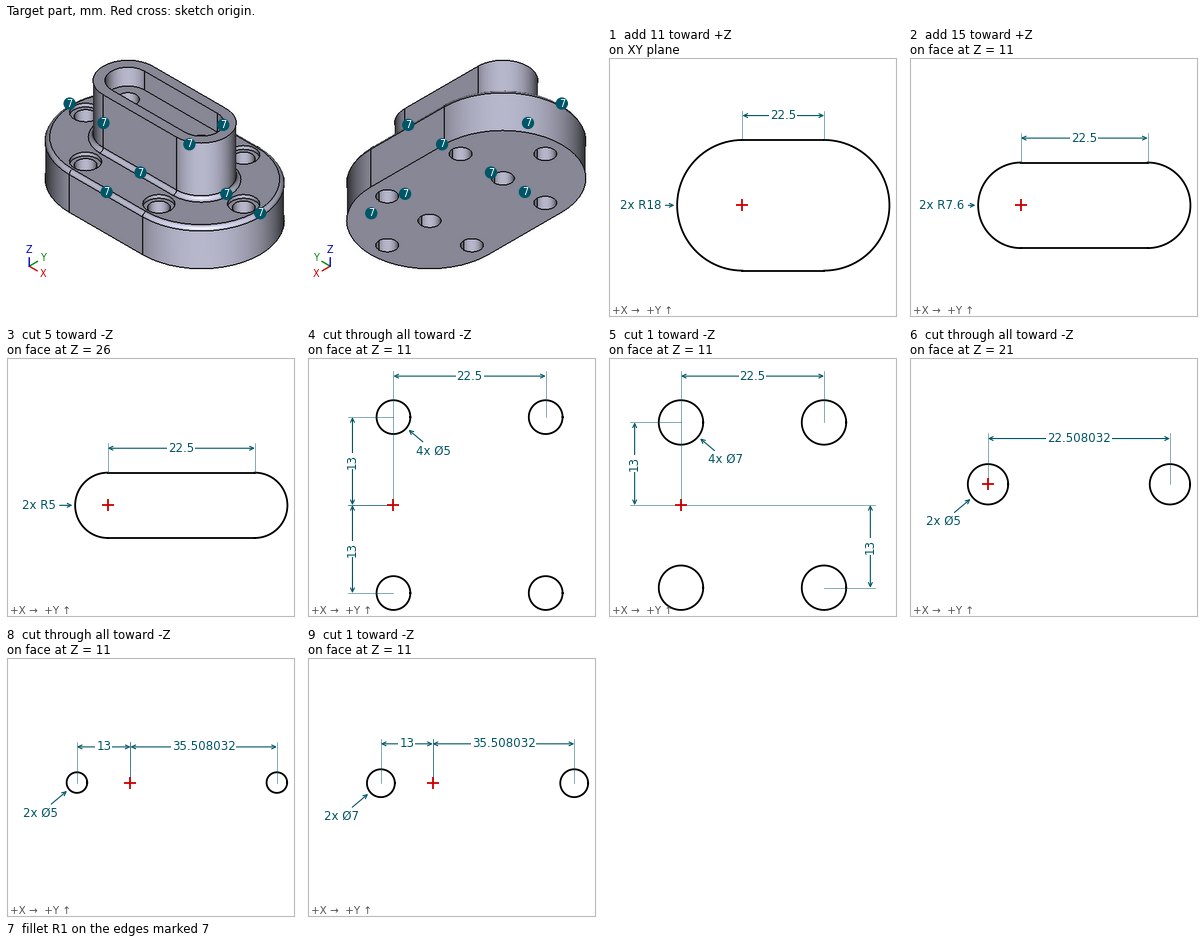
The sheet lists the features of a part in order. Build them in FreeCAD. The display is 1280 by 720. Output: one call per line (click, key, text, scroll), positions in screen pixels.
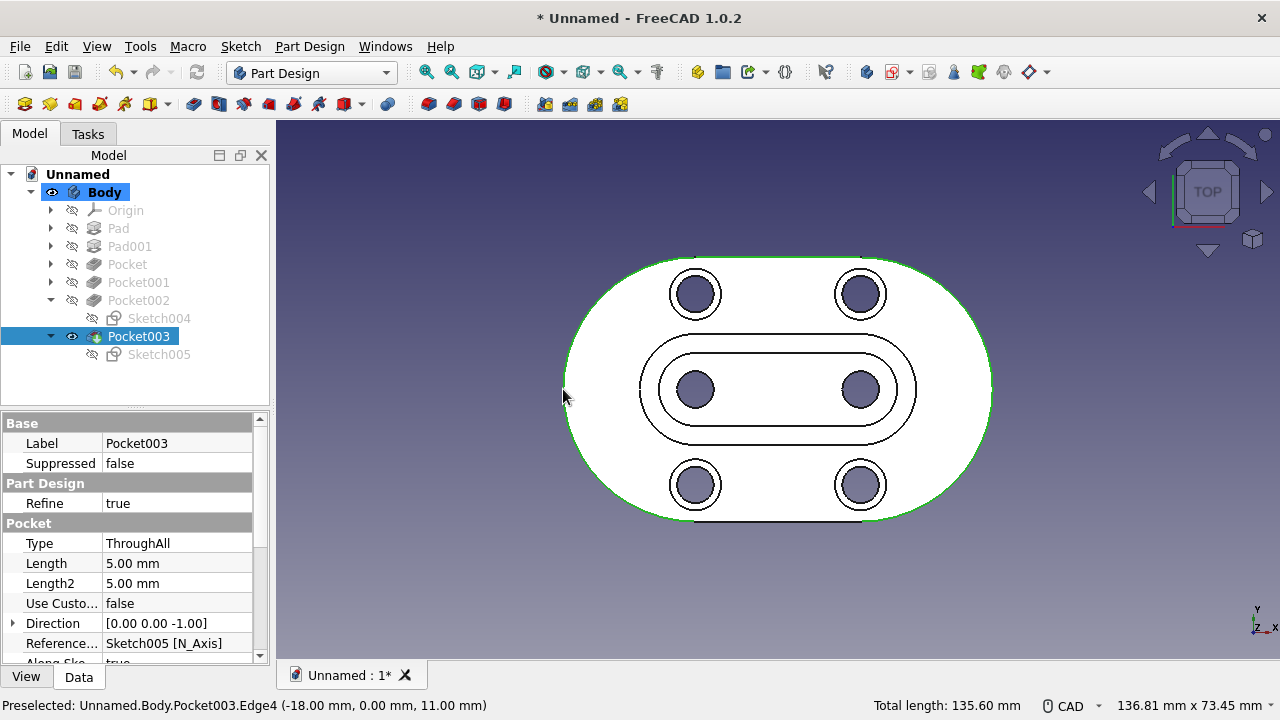
click(778, 521, ctrl)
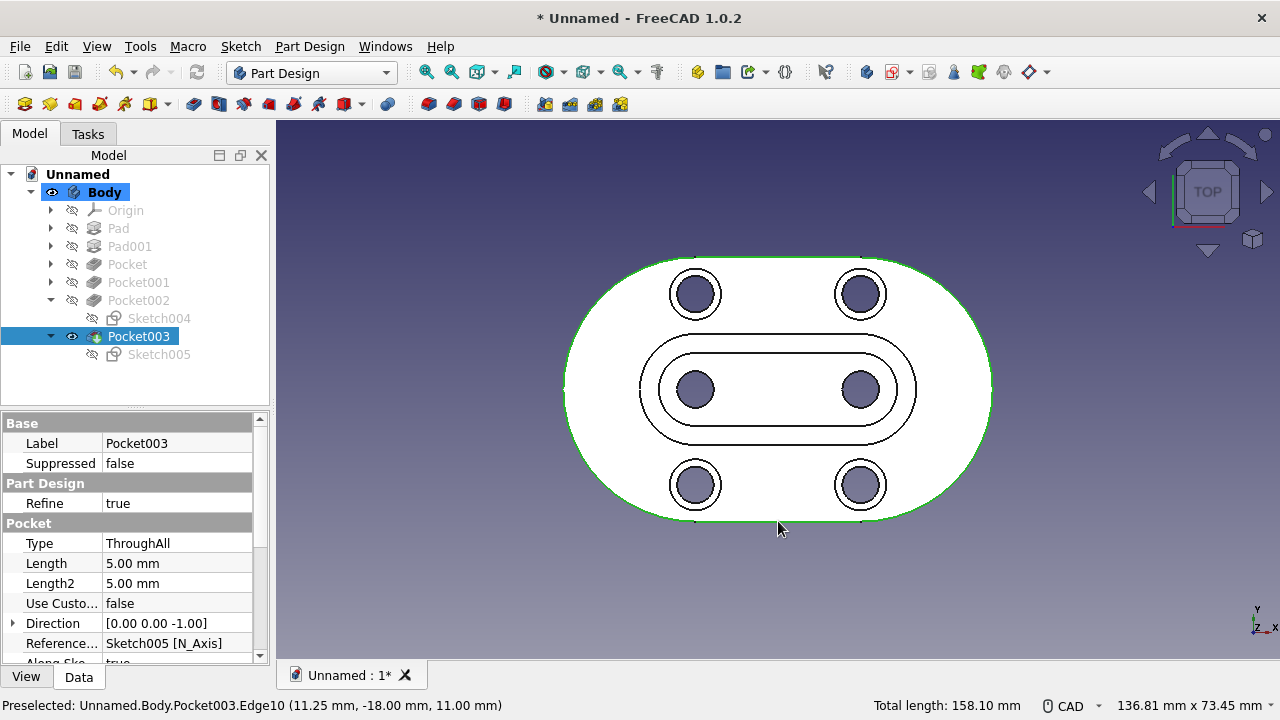
key(0)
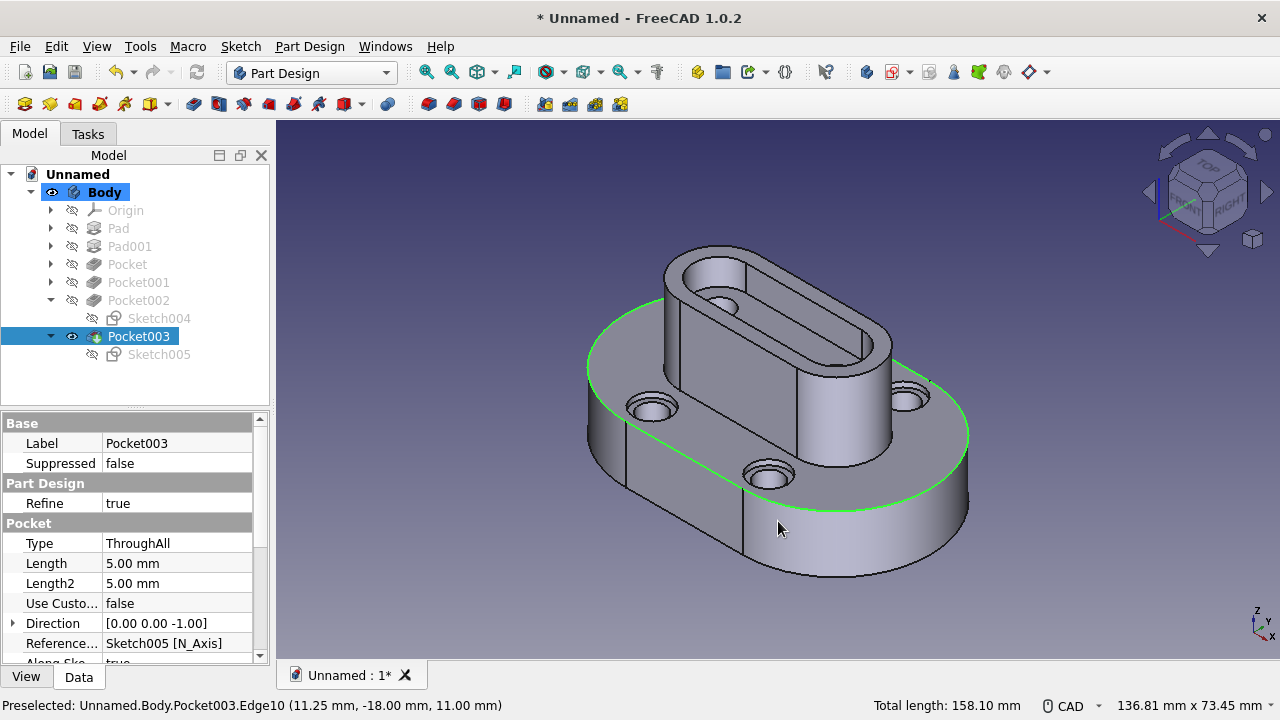
key(2)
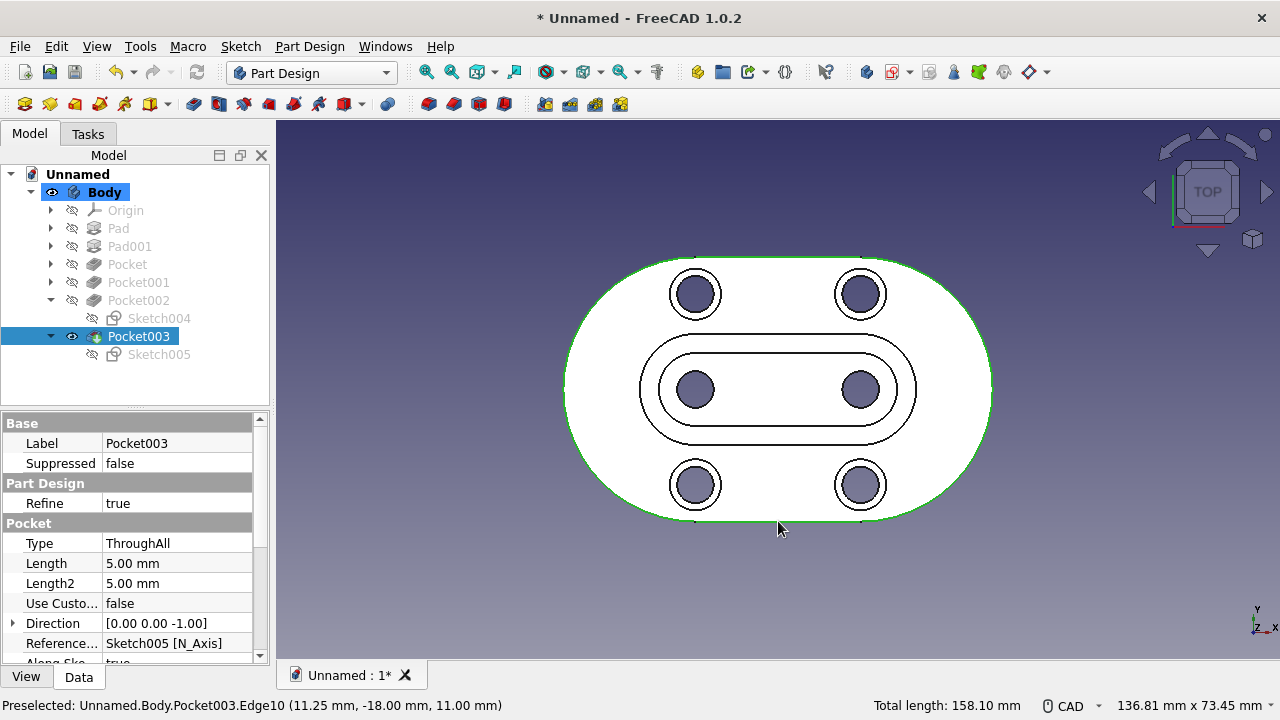
key(1)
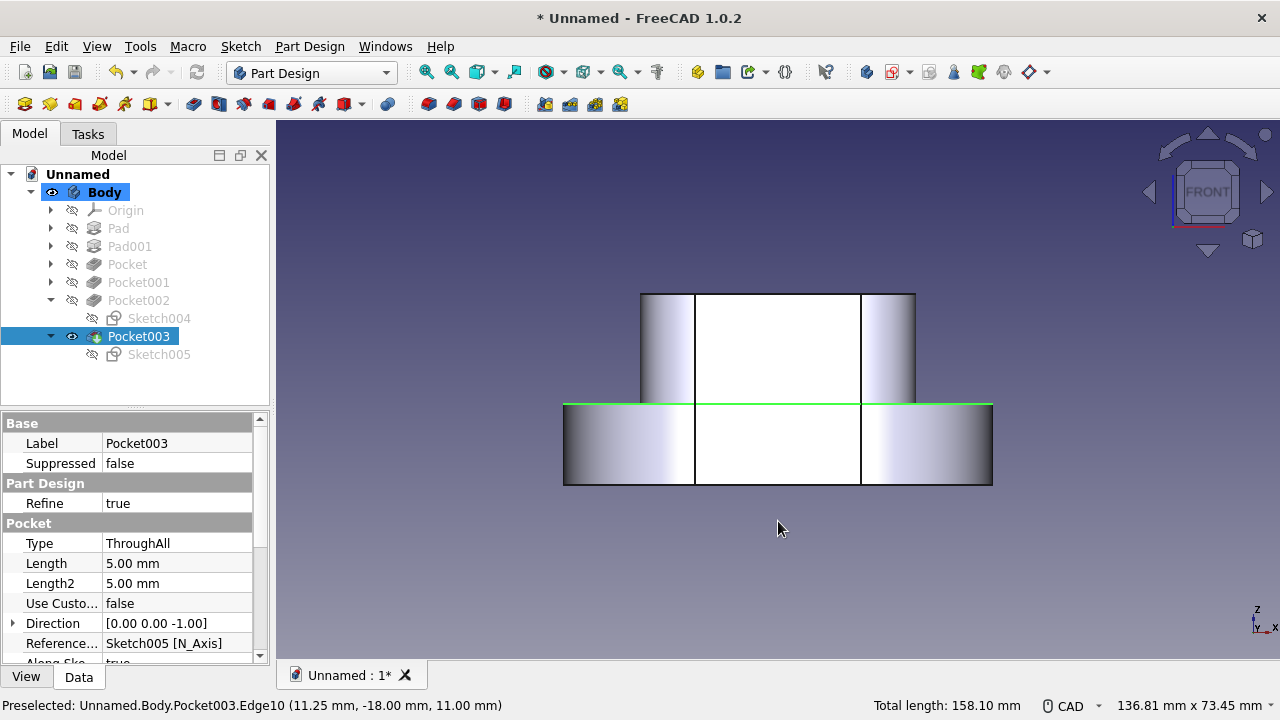
click(427, 72)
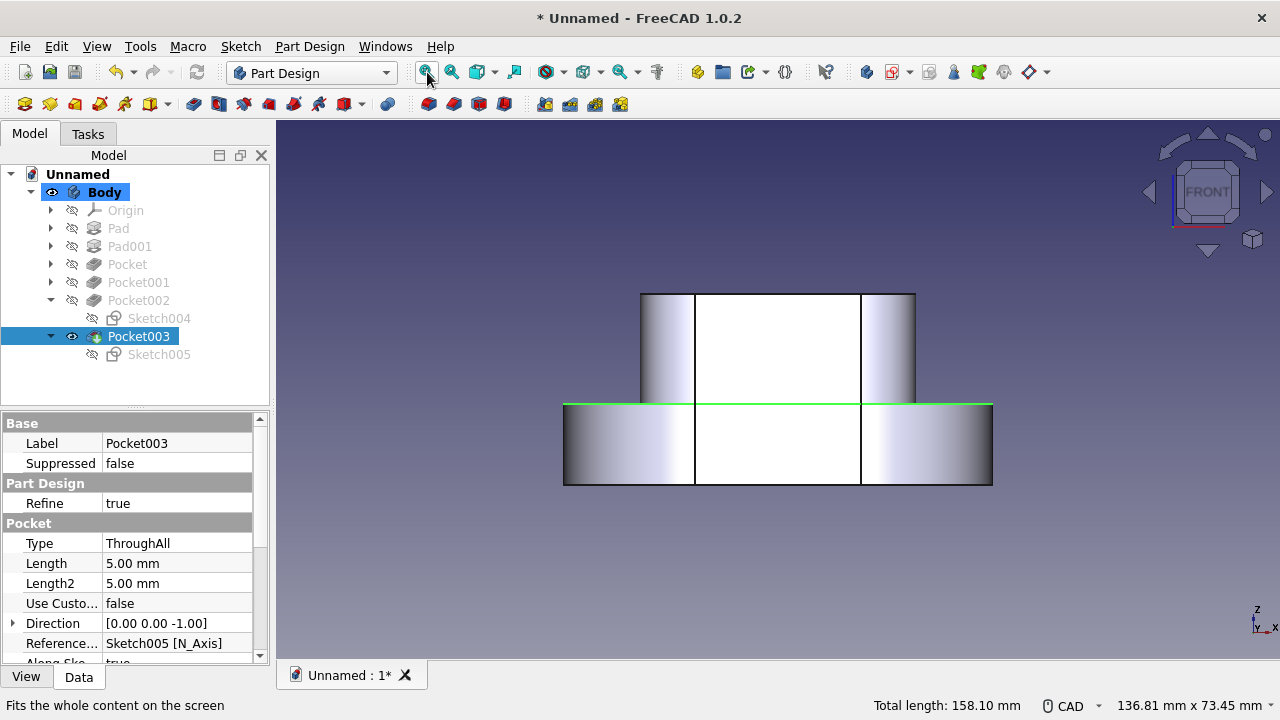
key(3)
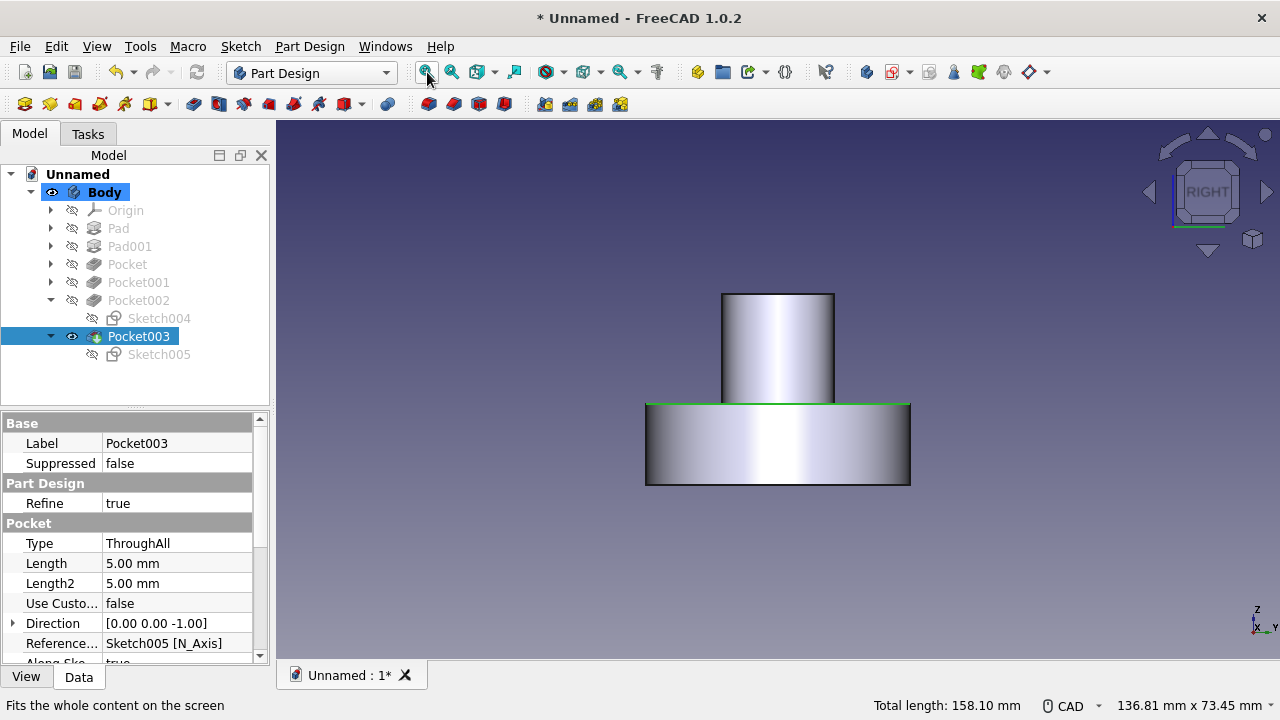
click(427, 72)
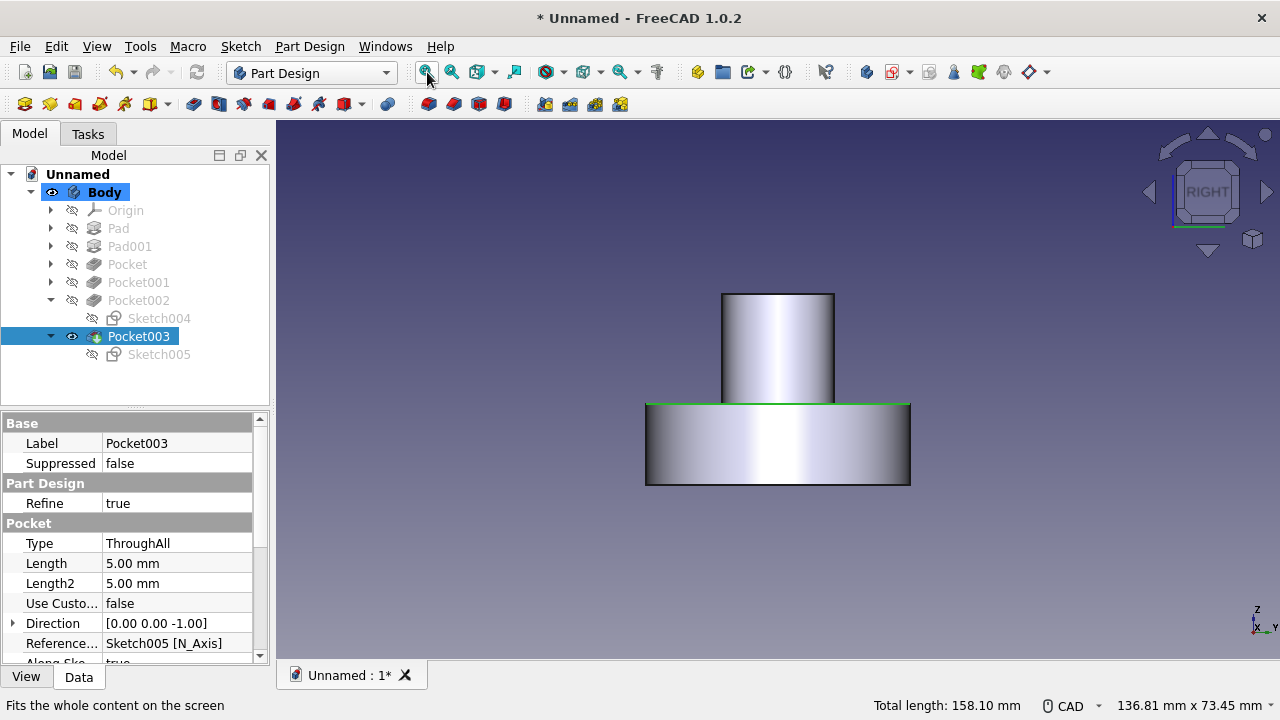
key(5)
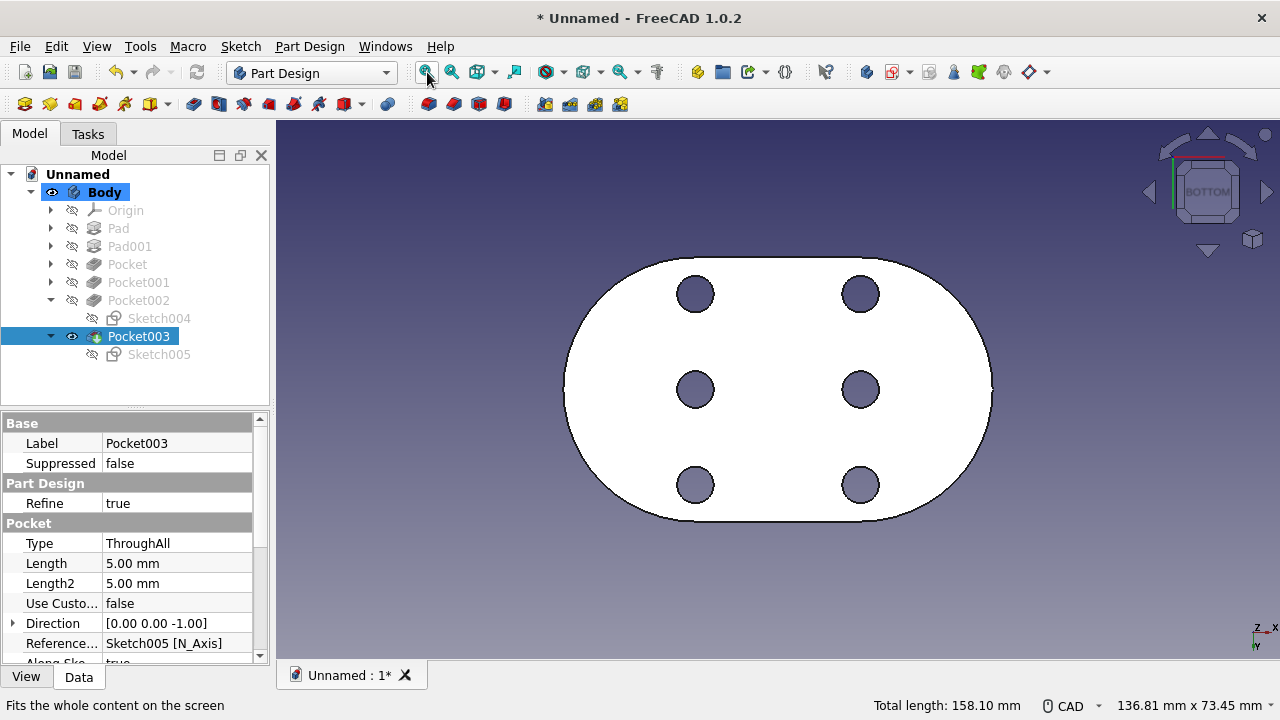
key(4)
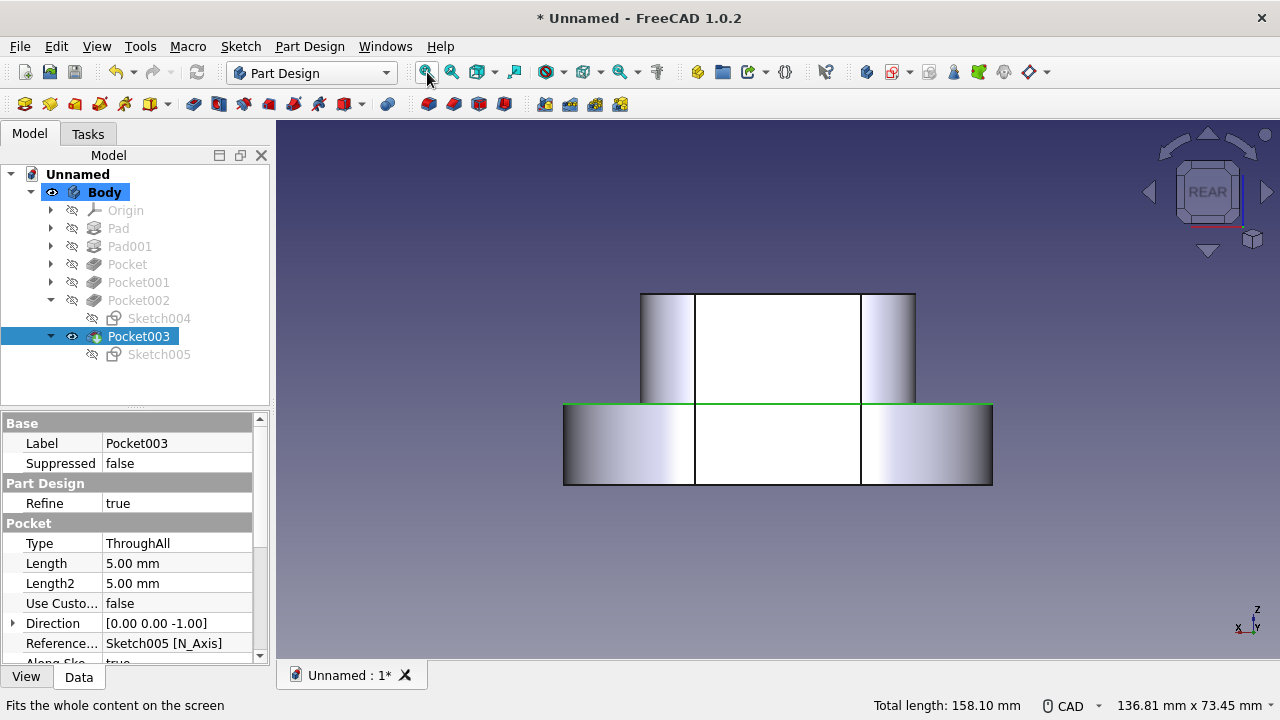
key(v)
key(f)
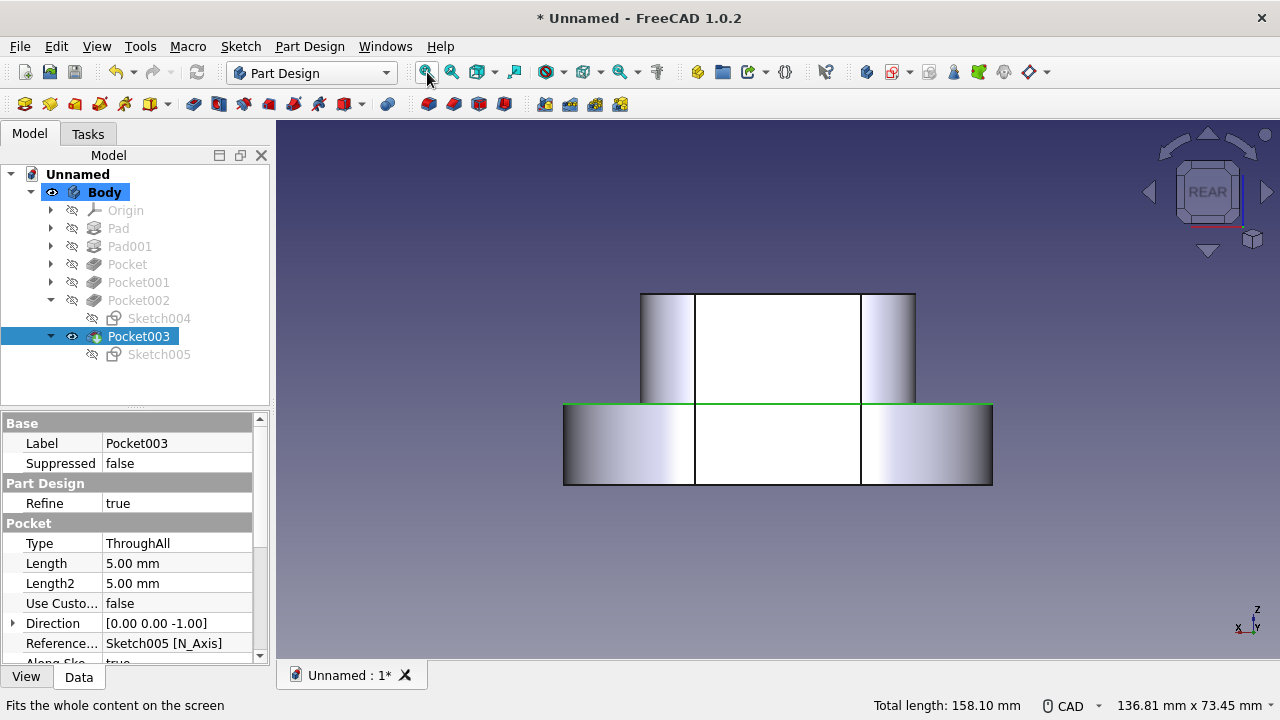
key(6)